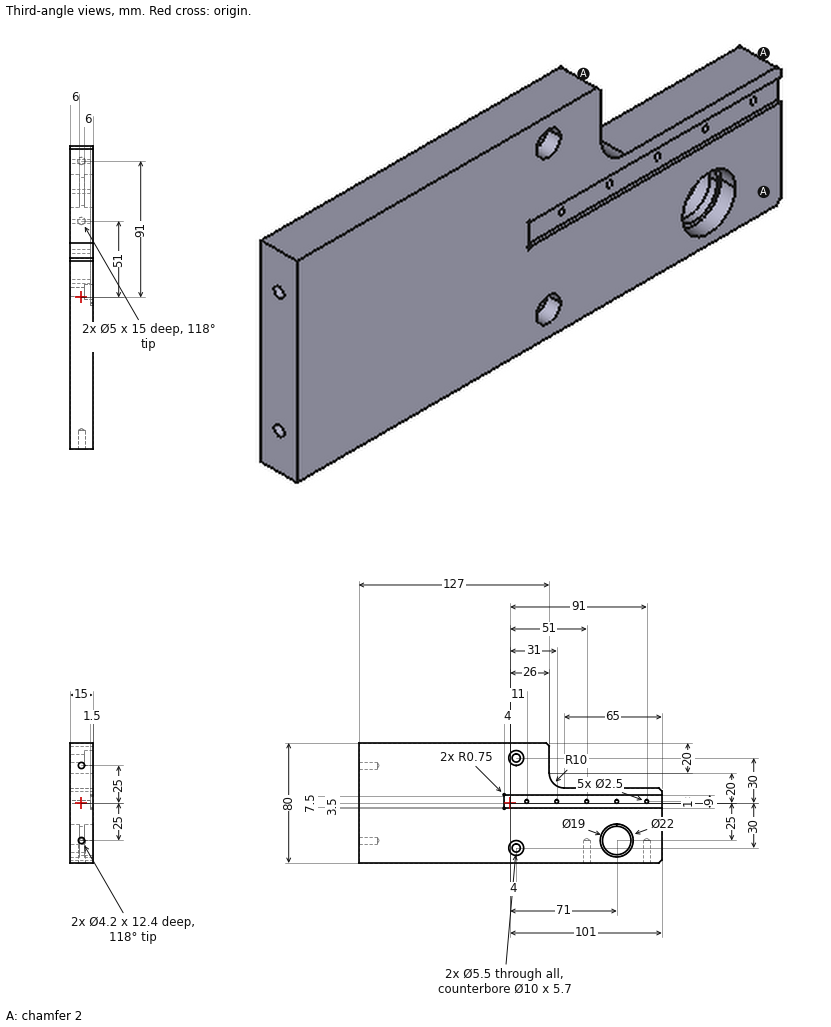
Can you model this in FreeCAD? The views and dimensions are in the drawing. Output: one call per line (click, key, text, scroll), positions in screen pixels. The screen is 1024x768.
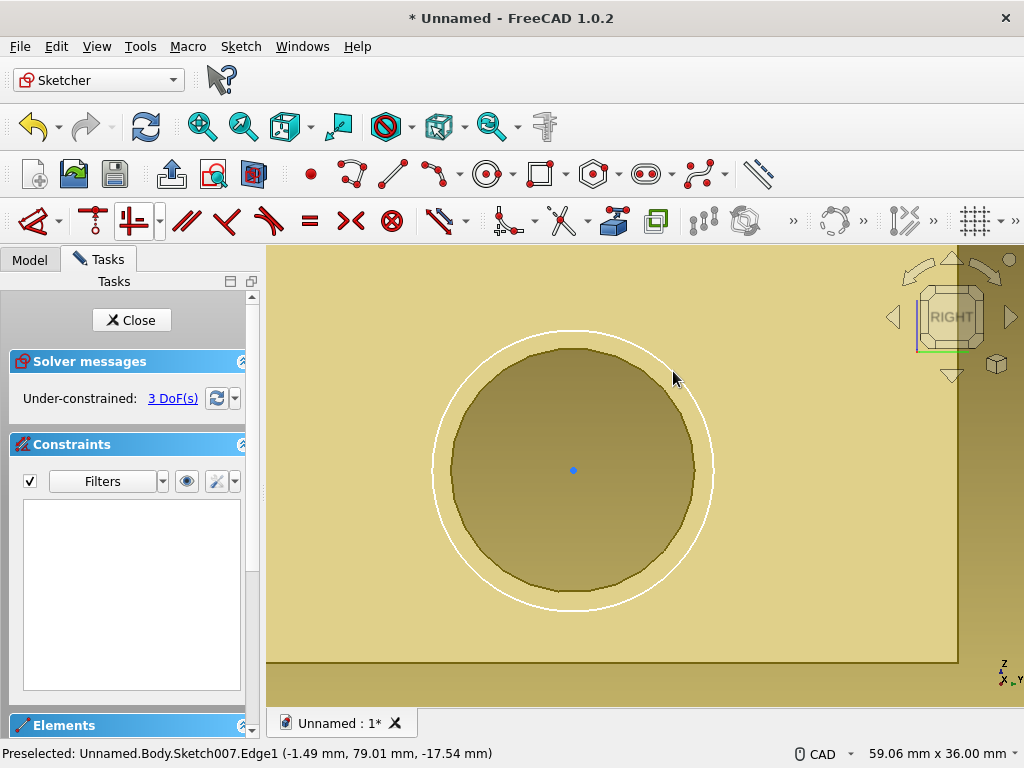
click(32, 222)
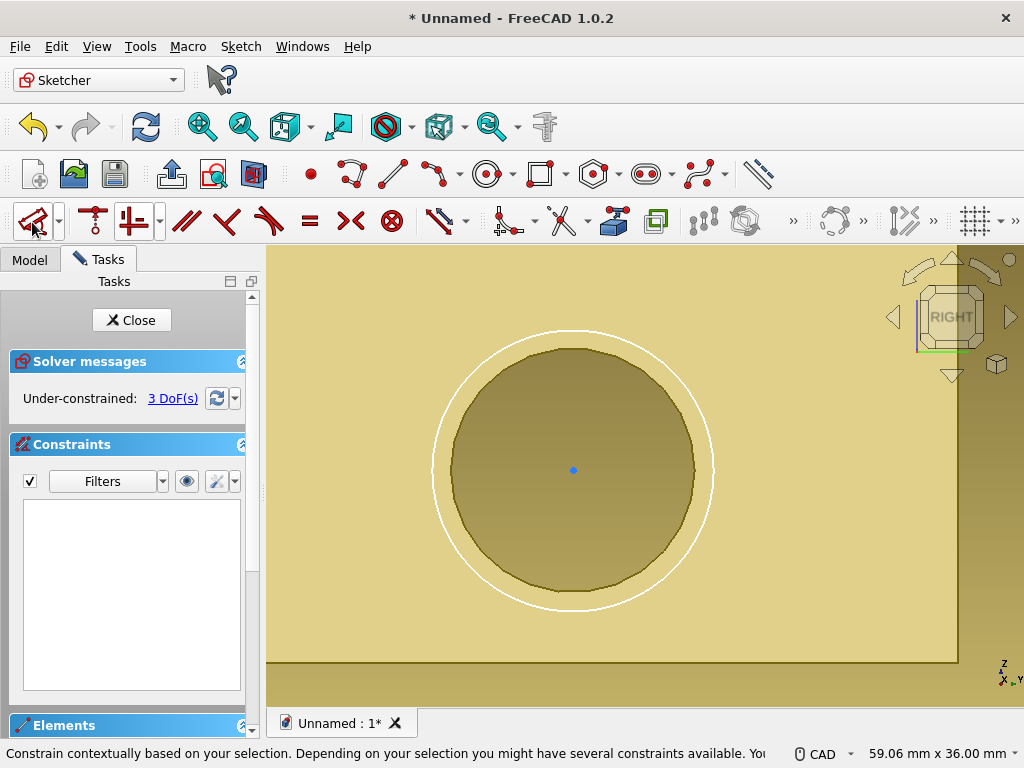
click(672, 371)
click(695, 348)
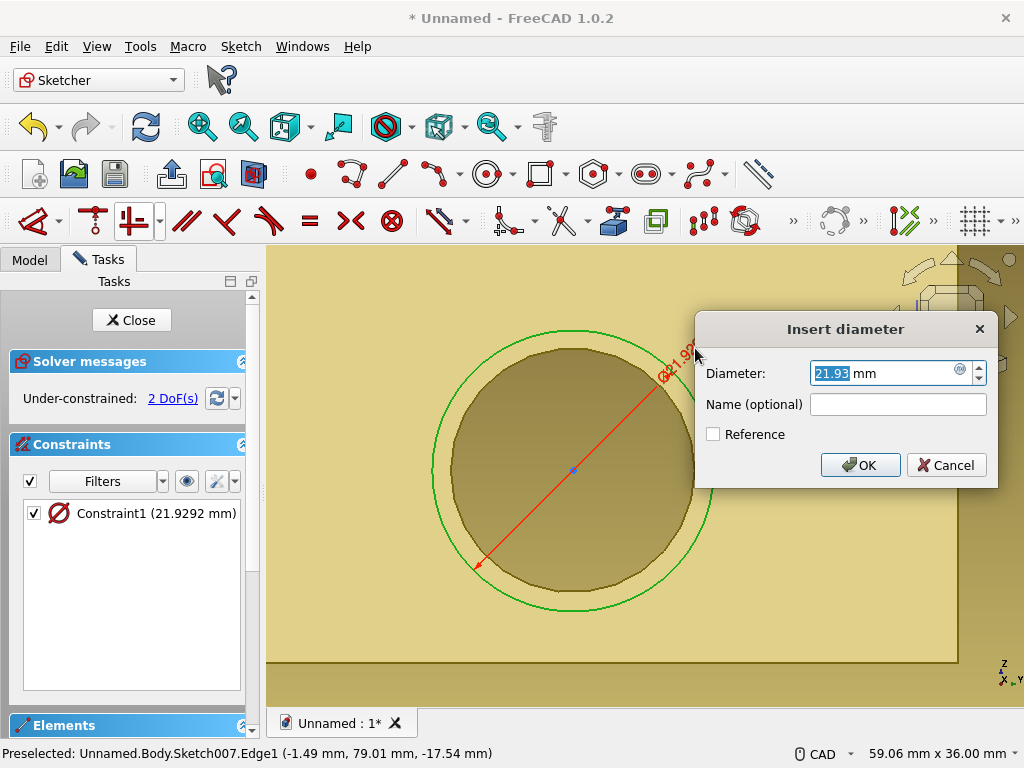
text(22)
key(Return)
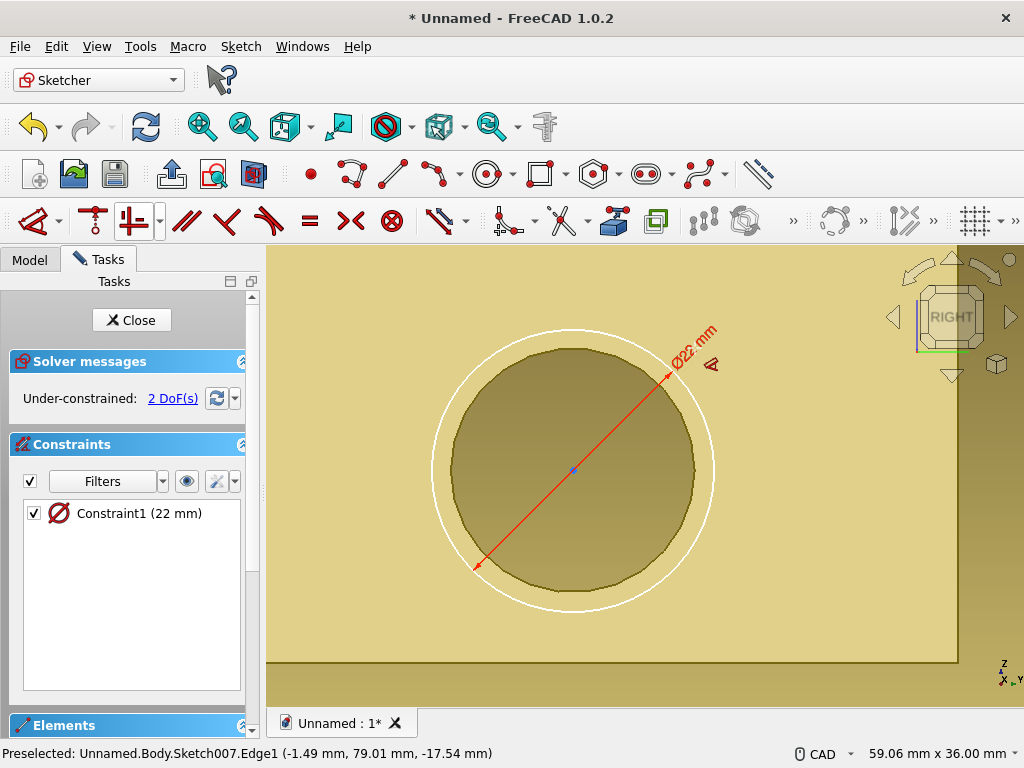
click(573, 471)
click(369, 505)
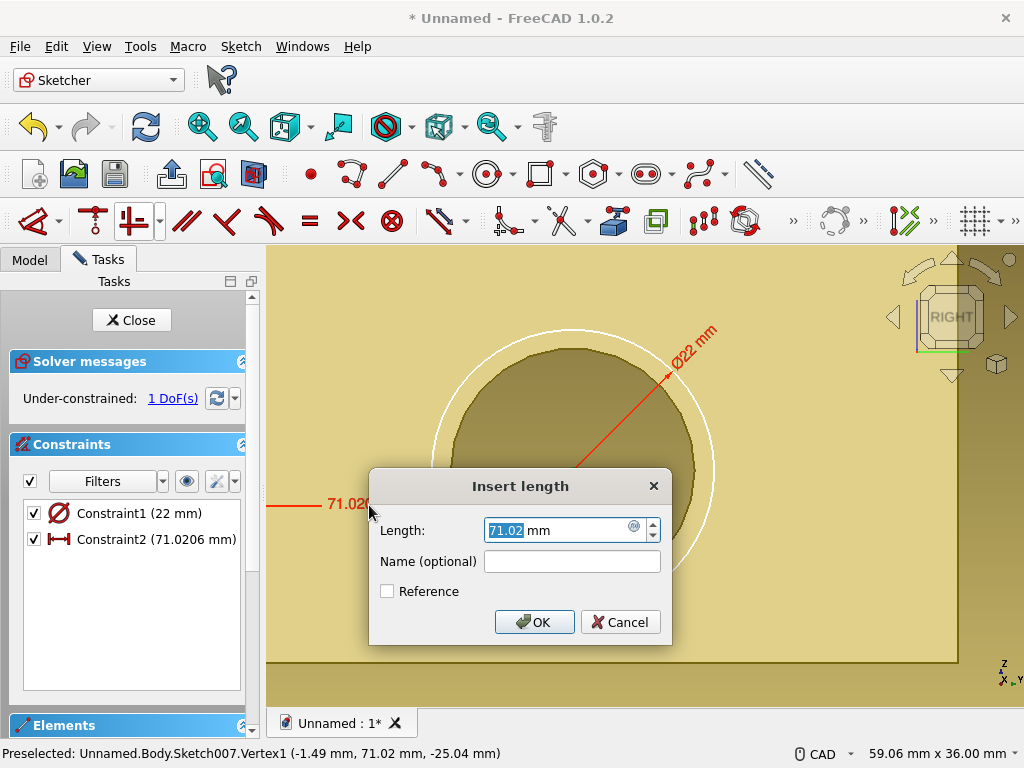
text(71)
key(Return)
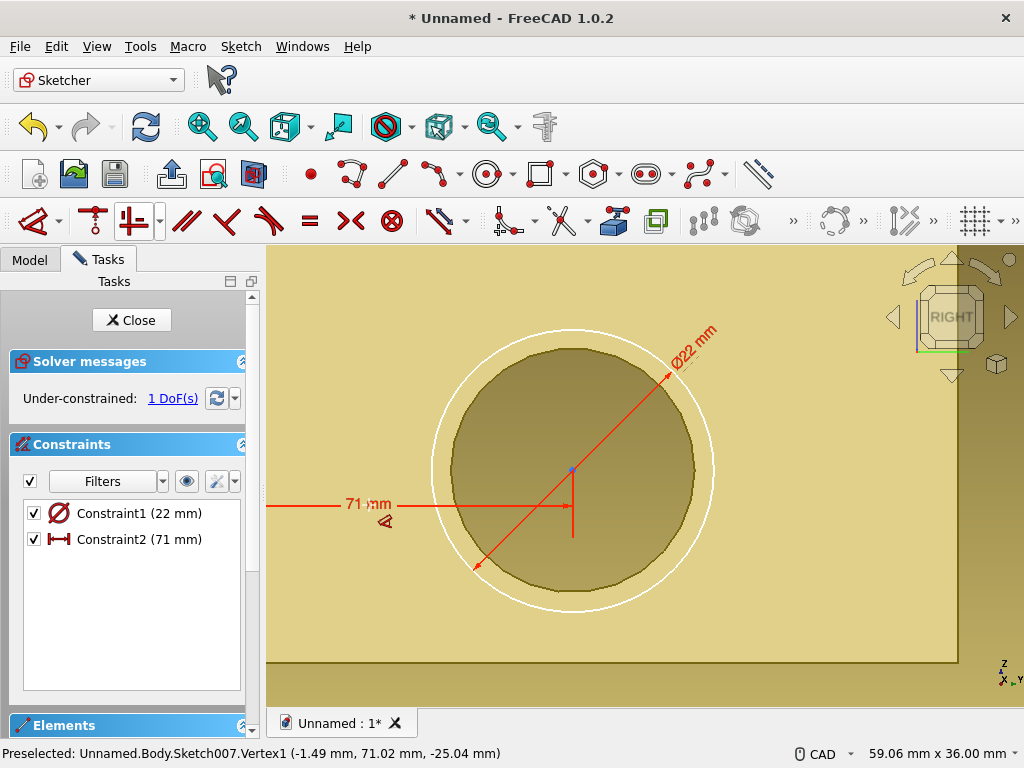
click(573, 471)
click(607, 372)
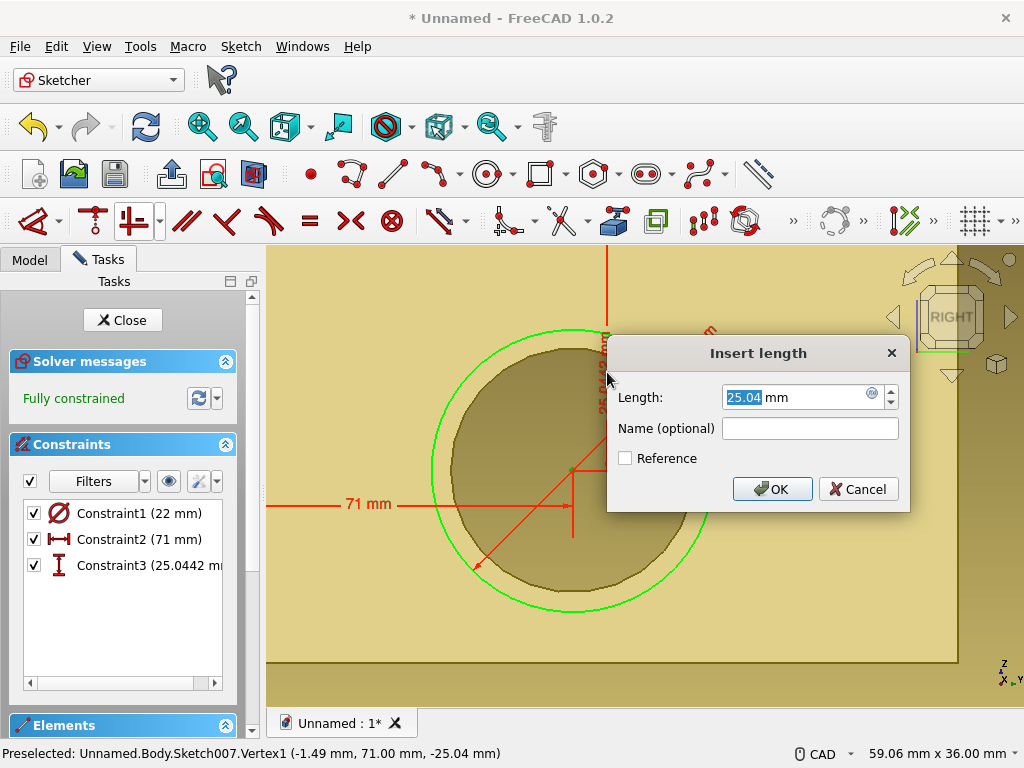
text(25)
key(Return)
key(Escape)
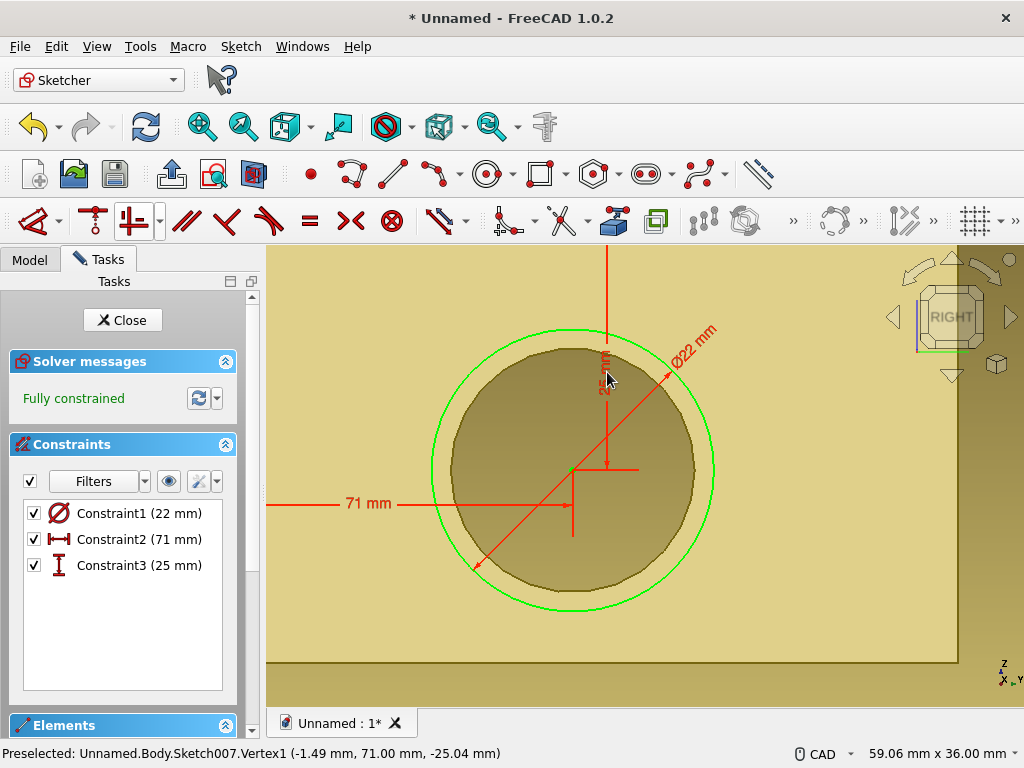
click(123, 320)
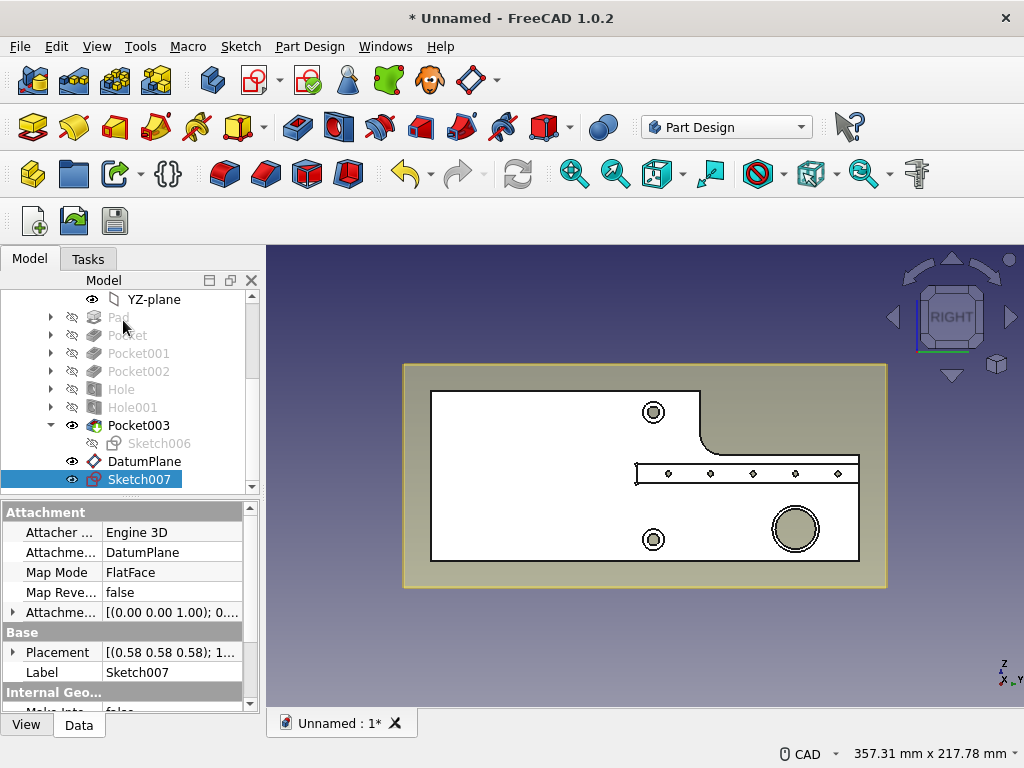
click(298, 128)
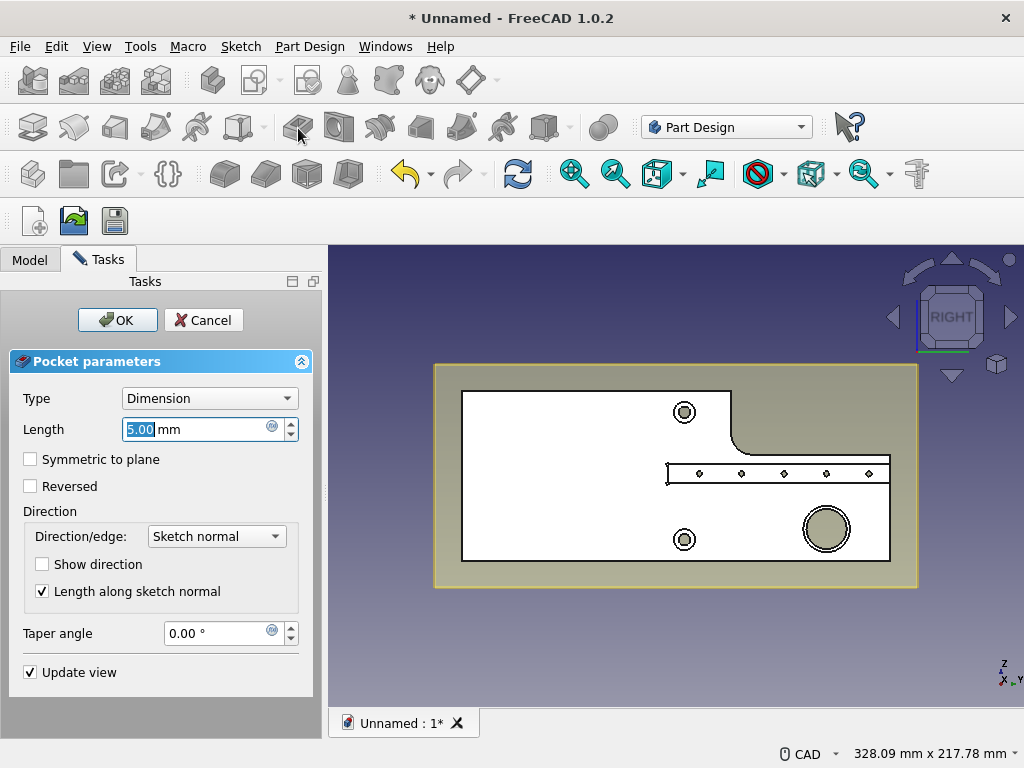
text(6)
key(Tab)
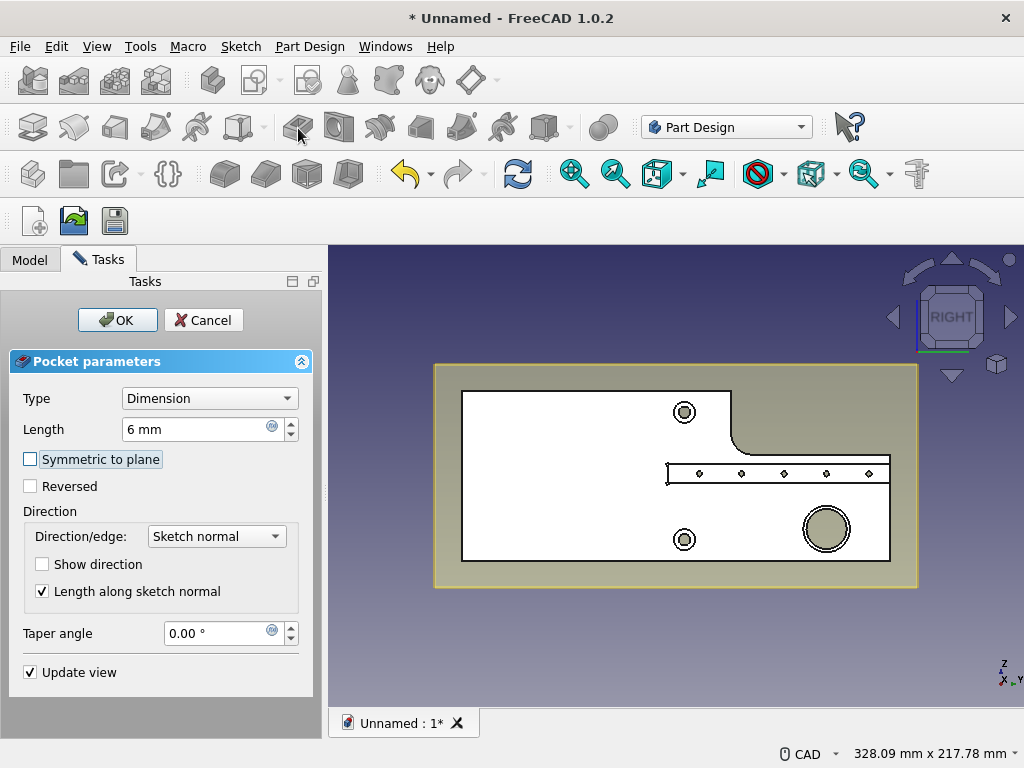
click(118, 320)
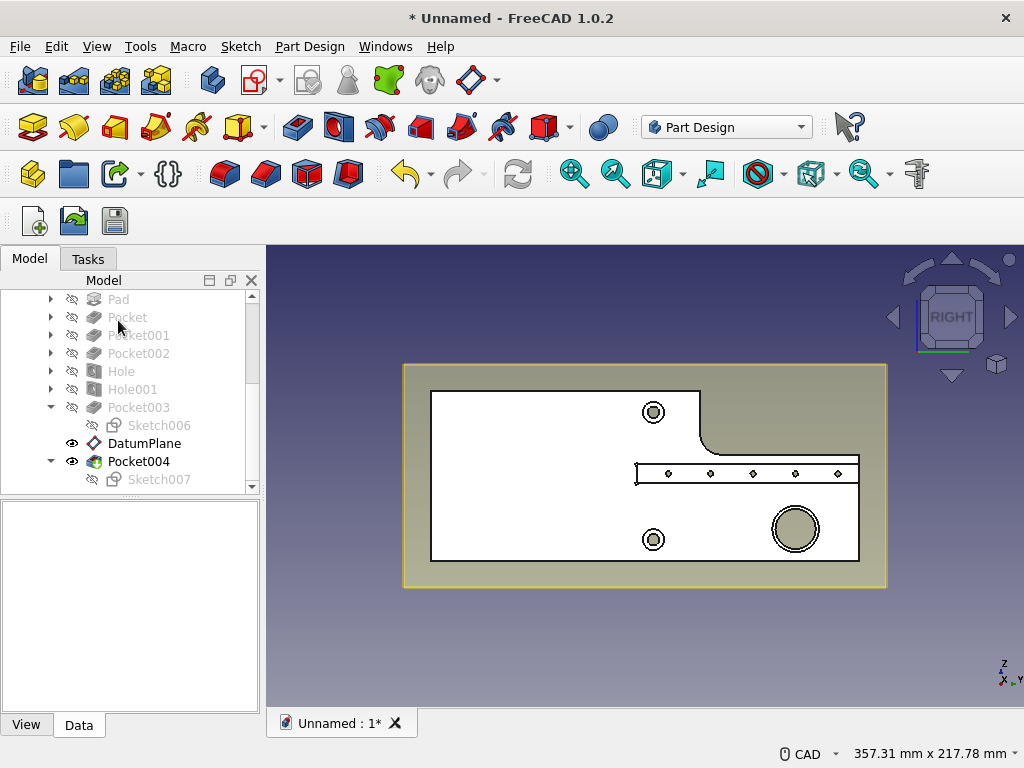
click(117, 443)
key(space)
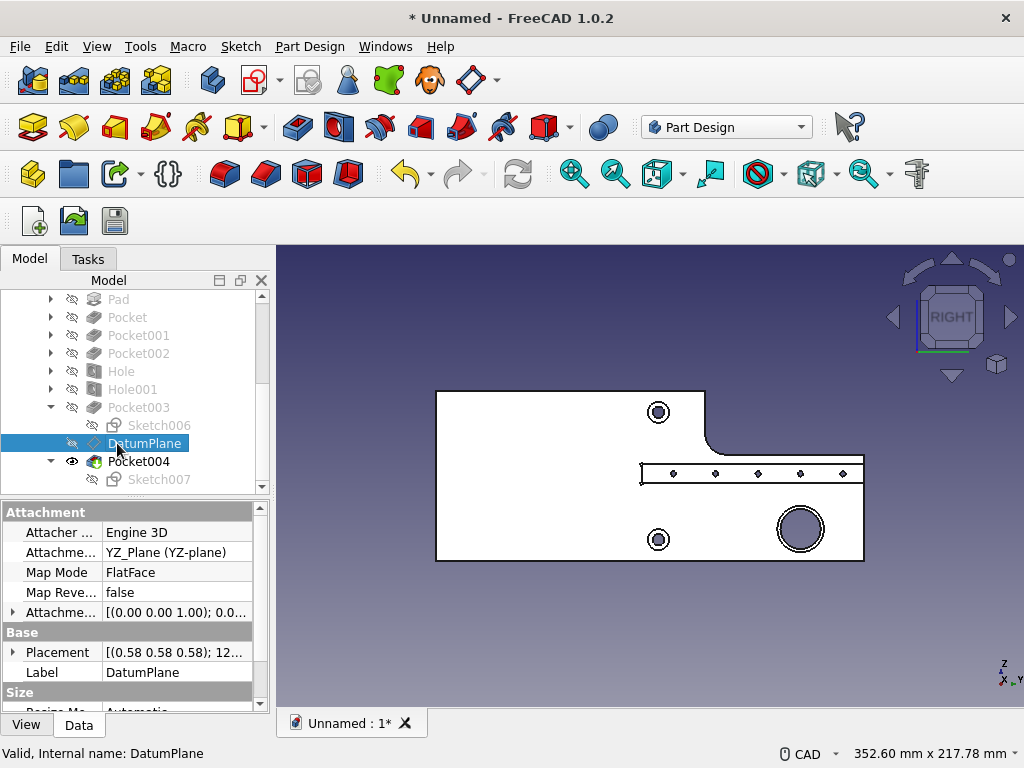
key(5)